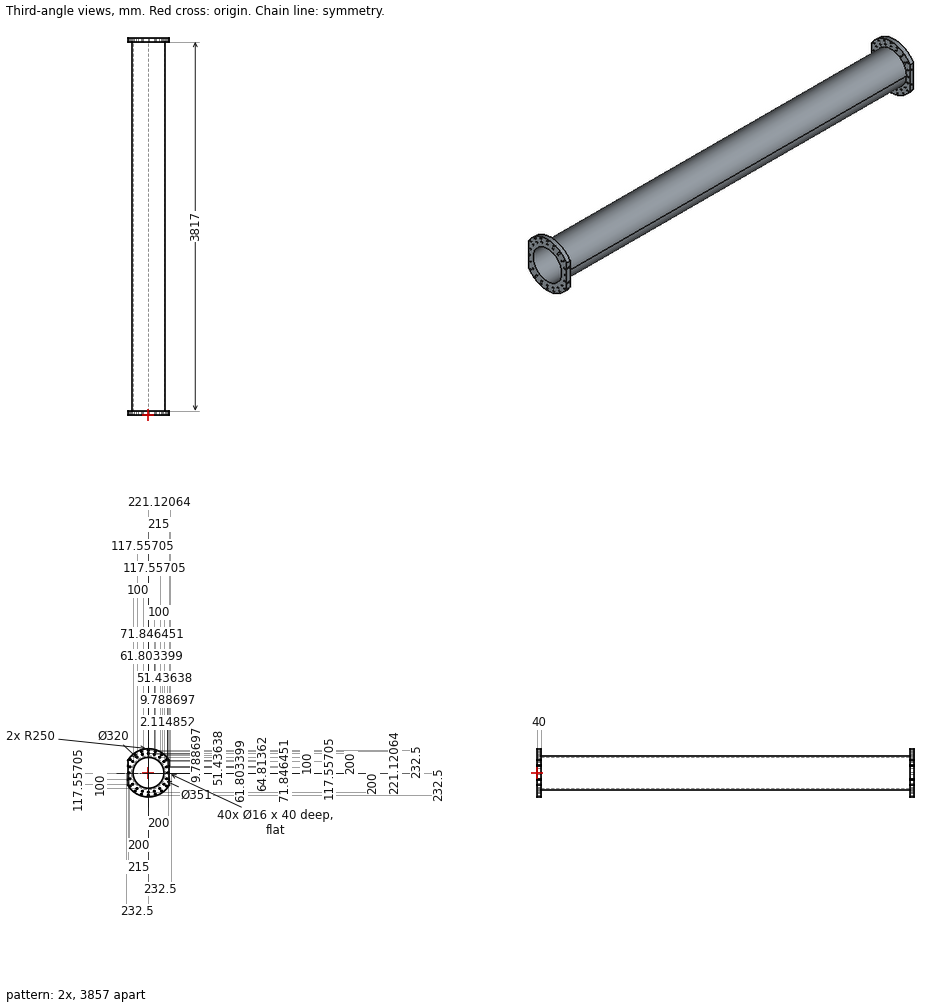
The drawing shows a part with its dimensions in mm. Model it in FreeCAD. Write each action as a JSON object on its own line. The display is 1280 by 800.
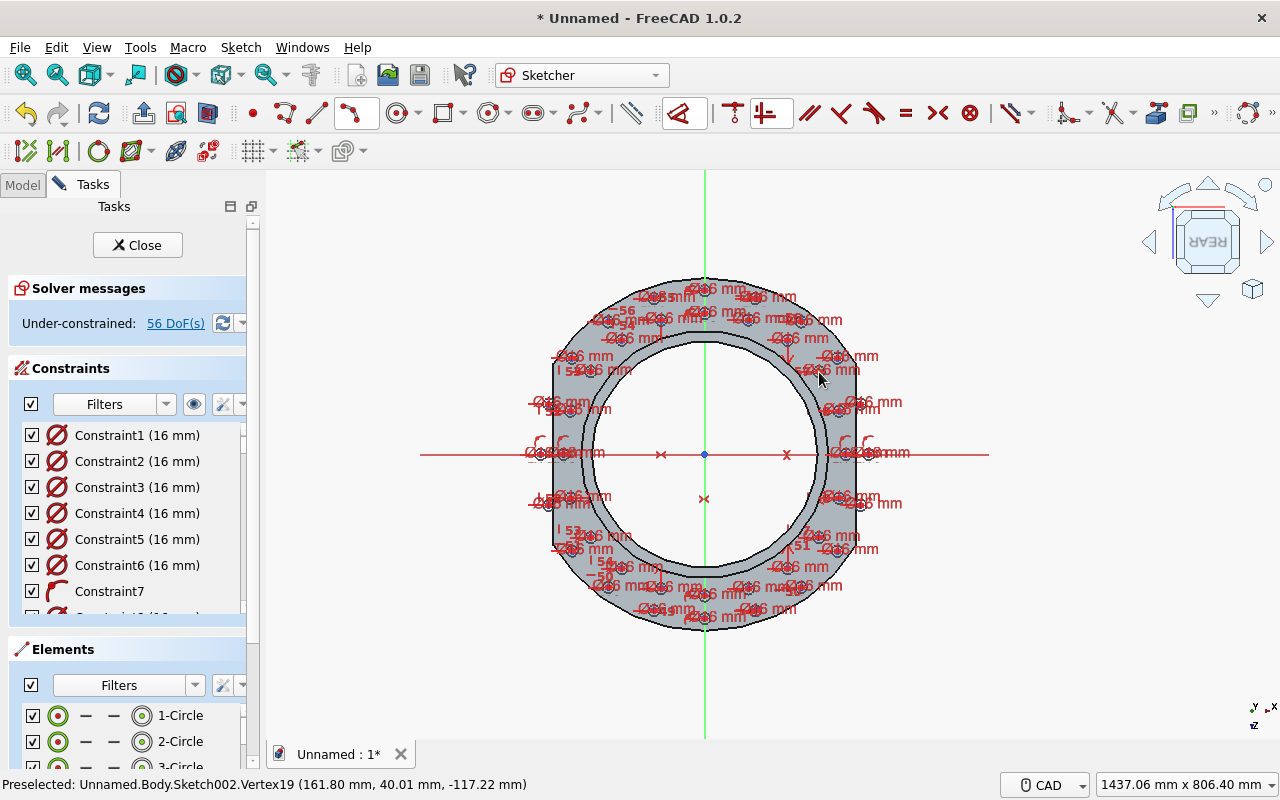
{"action": "left_click", "coordinate": [705, 674]}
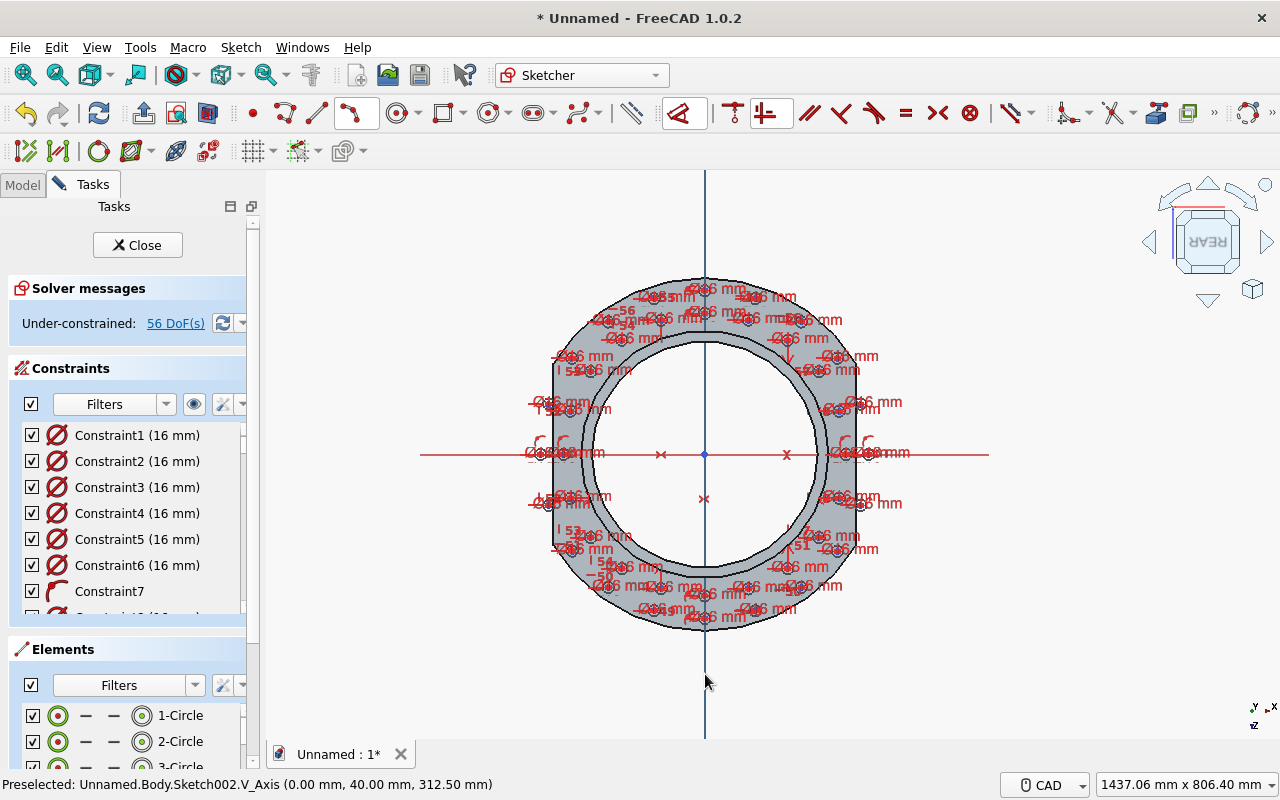
{"action": "left_click", "coordinate": [938, 114]}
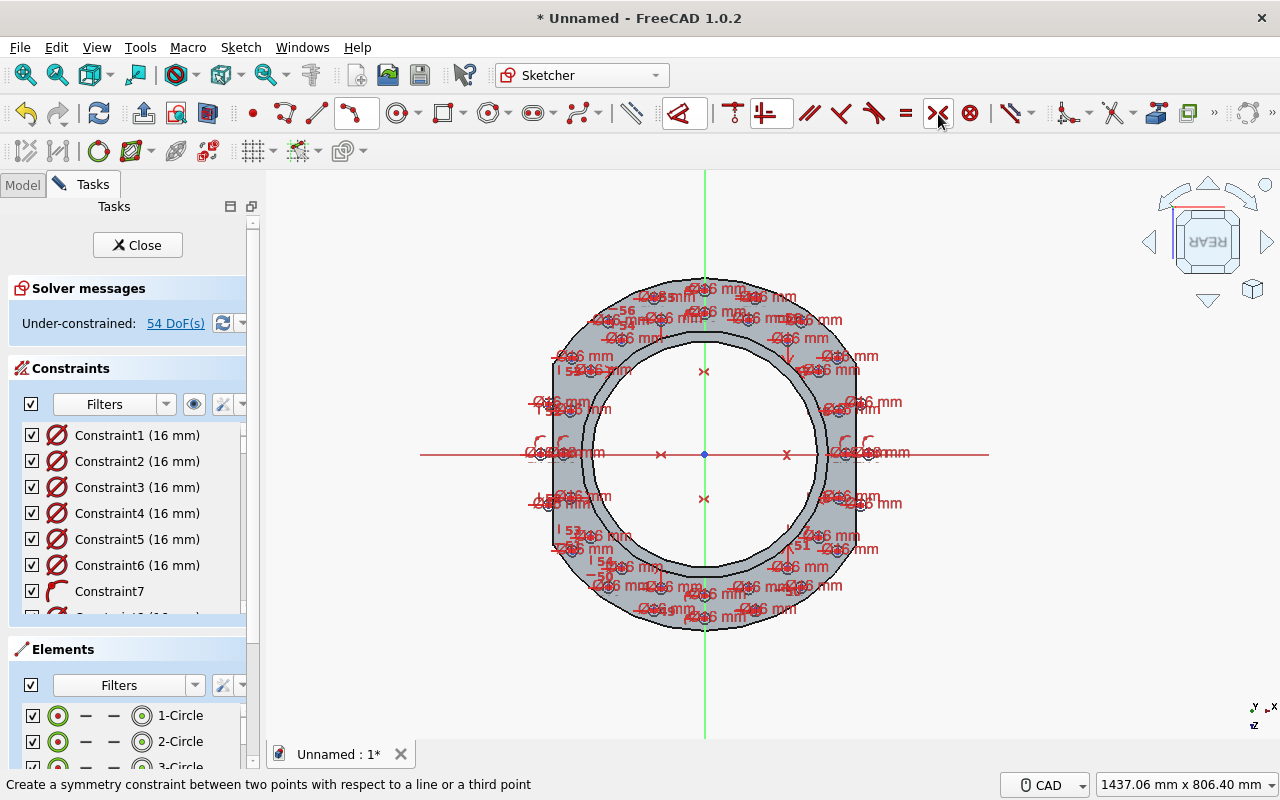
{"action": "left_click", "coordinate": [755, 611]}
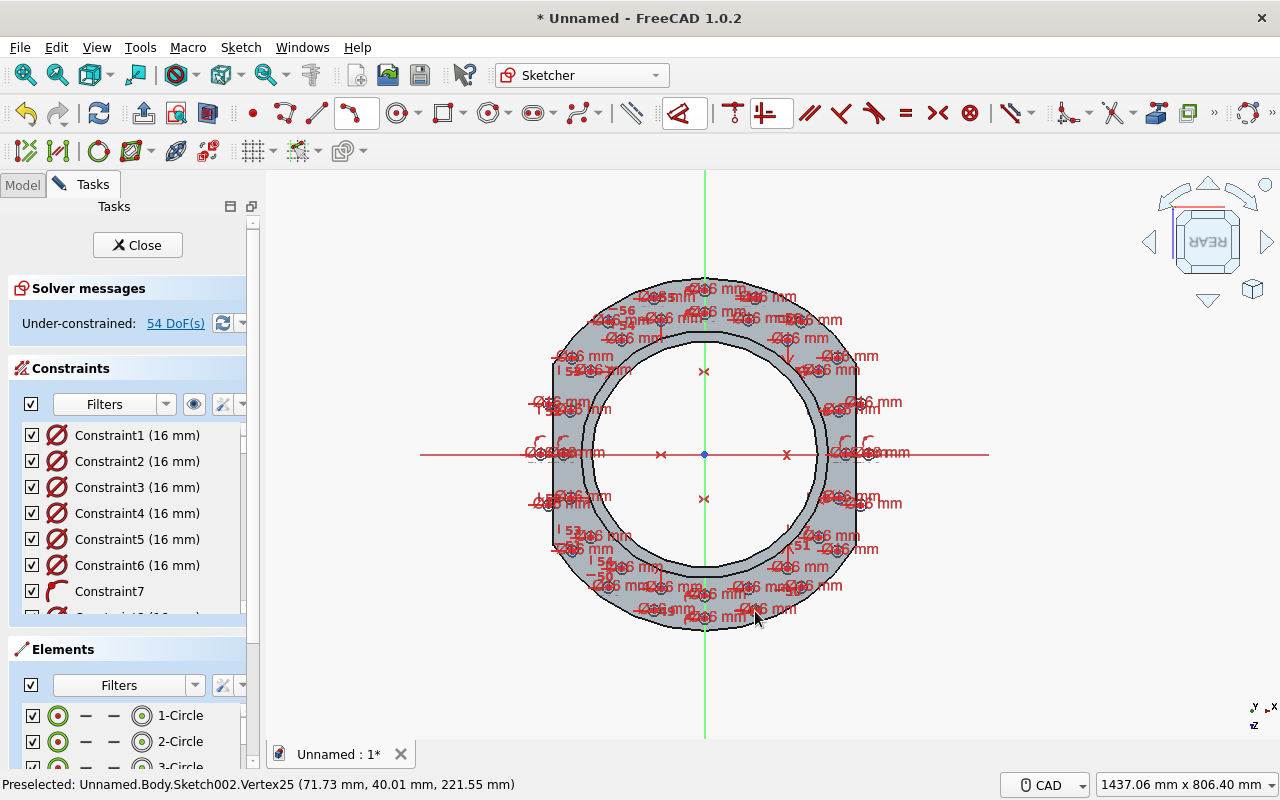
{"action": "scroll", "coordinate": [654, 611], "scroll_direction": "up", "scroll_amount": 4}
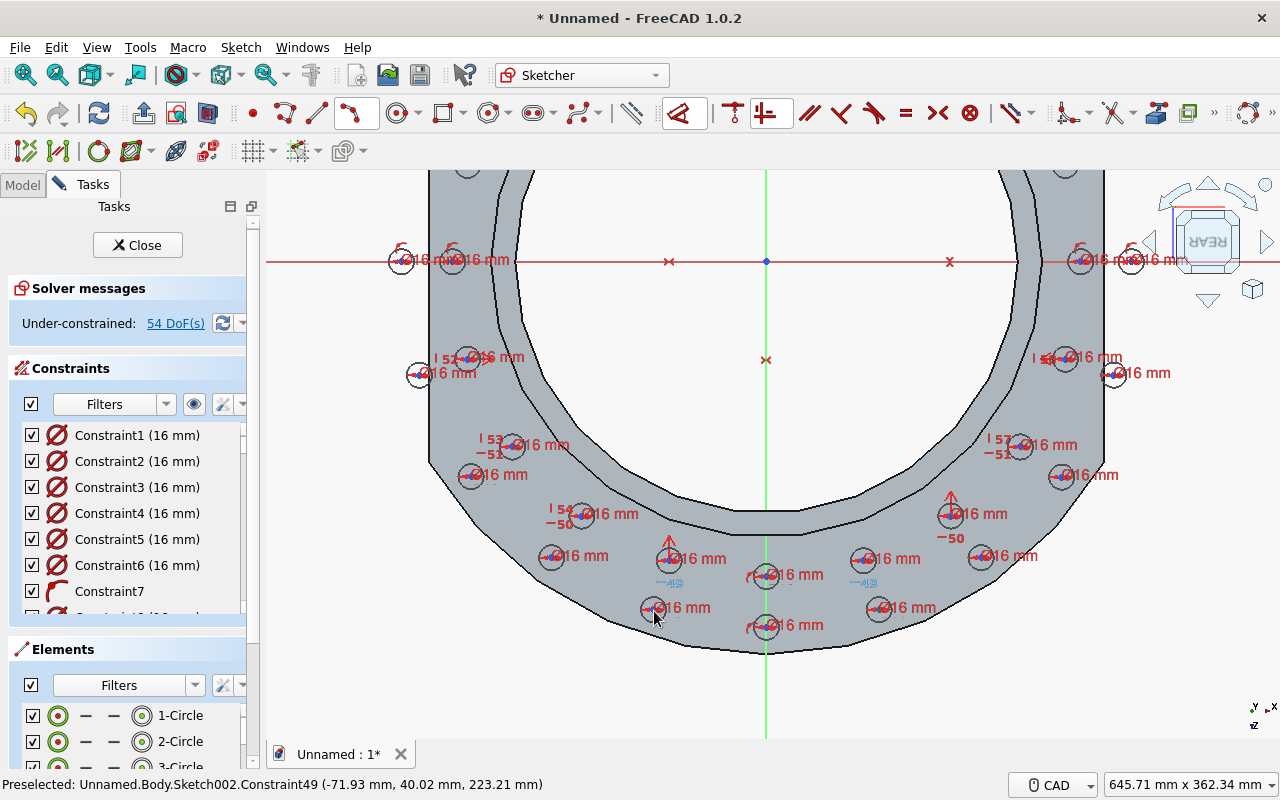
{"action": "left_click", "coordinate": [654, 610]}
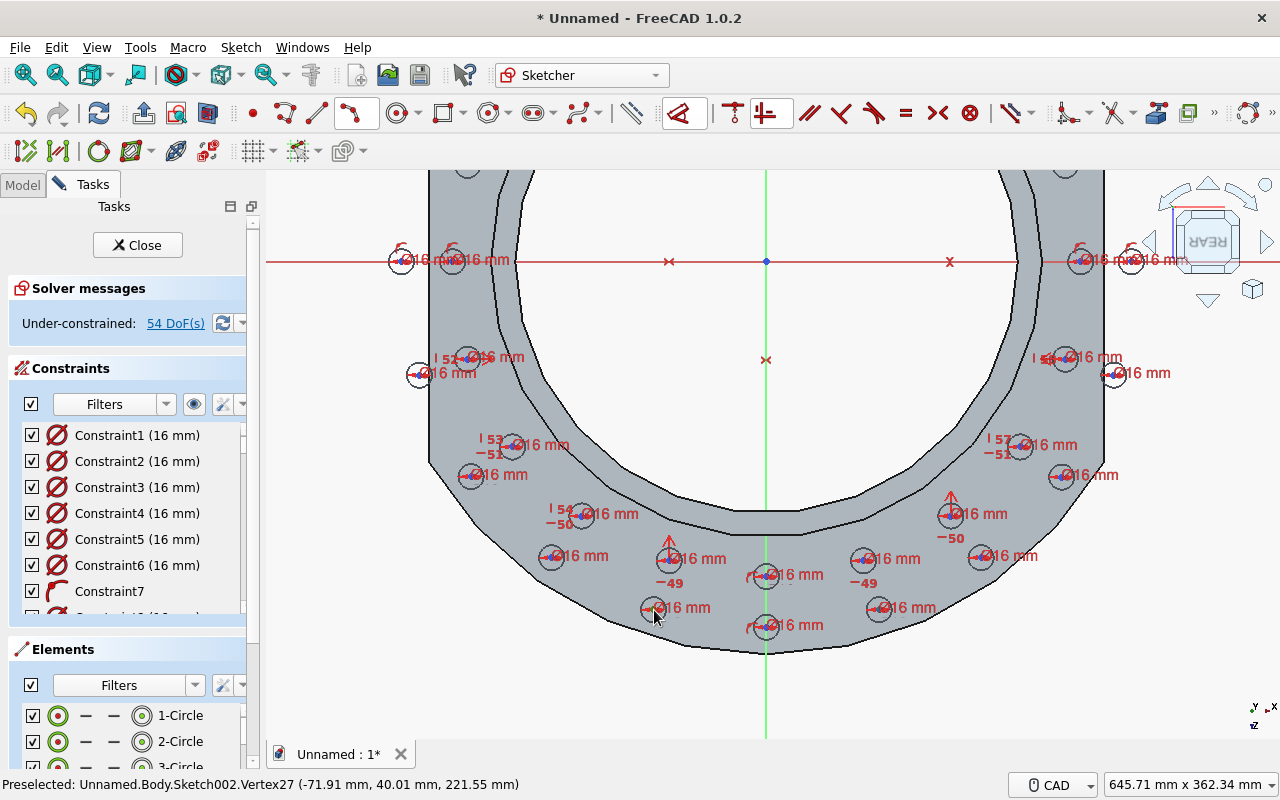
{"action": "left_click", "coordinate": [766, 674]}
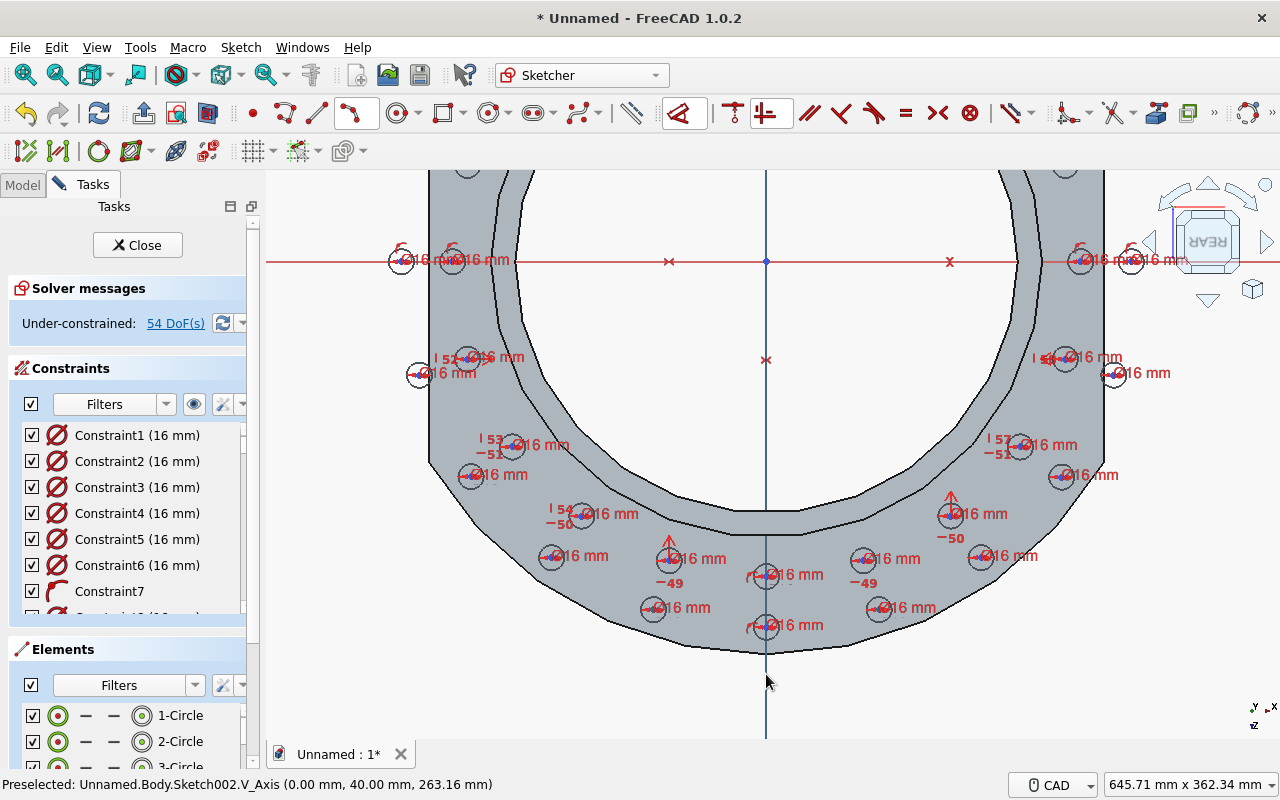
{"action": "left_click", "coordinate": [938, 114]}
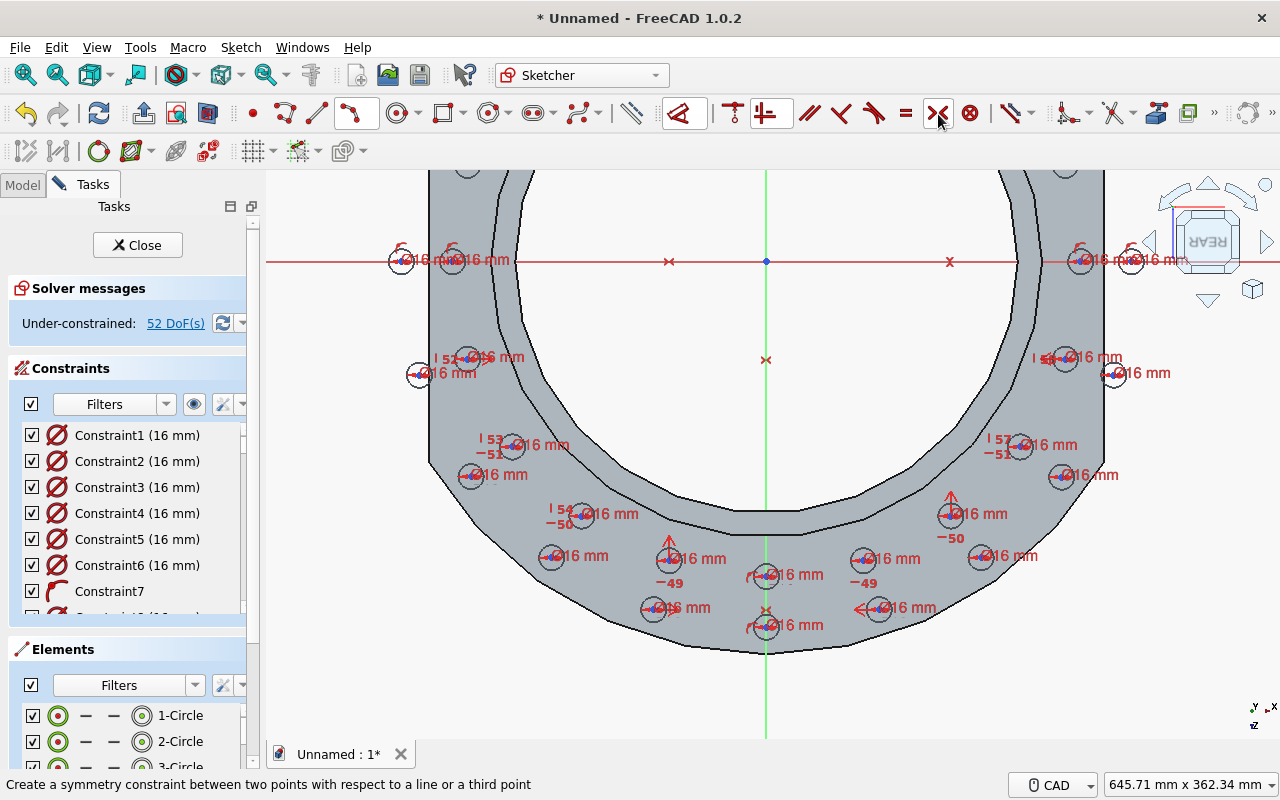
{"action": "left_click", "coordinate": [981, 558]}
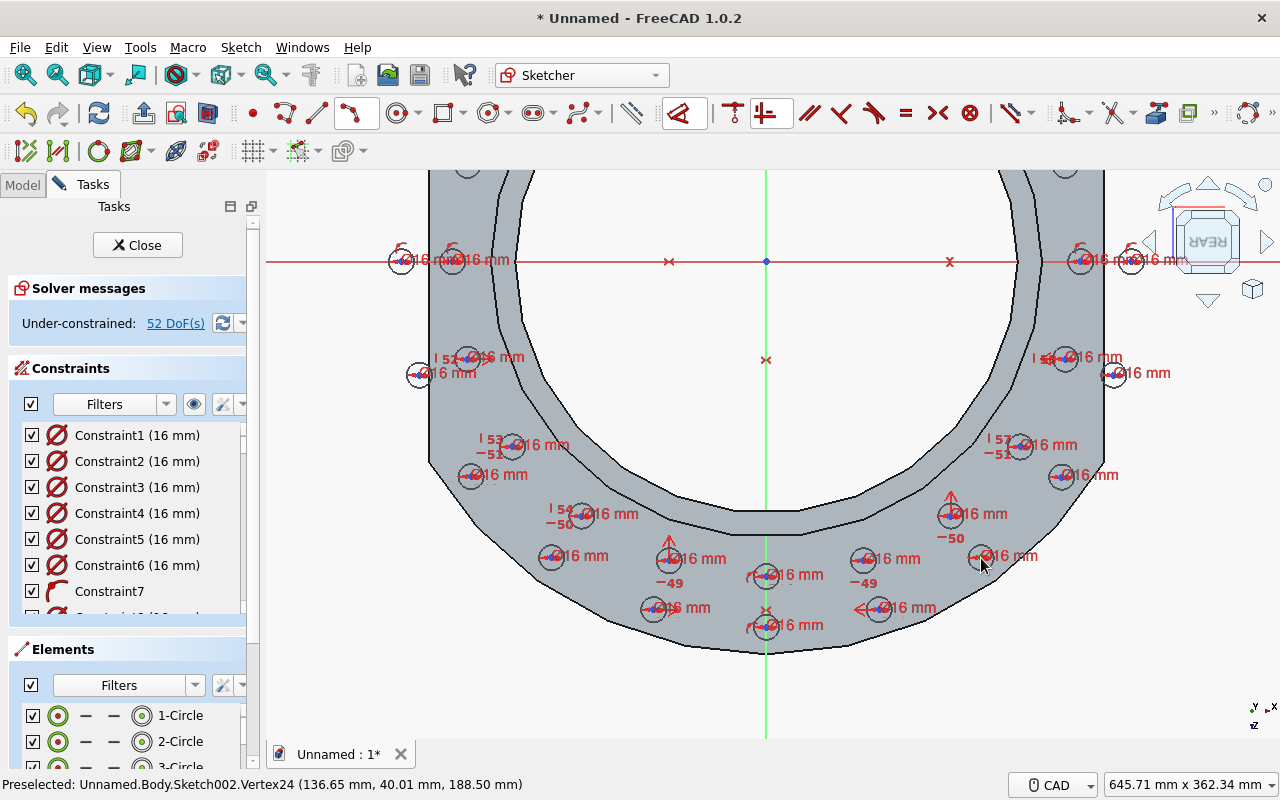
{"action": "left_click", "coordinate": [552, 558]}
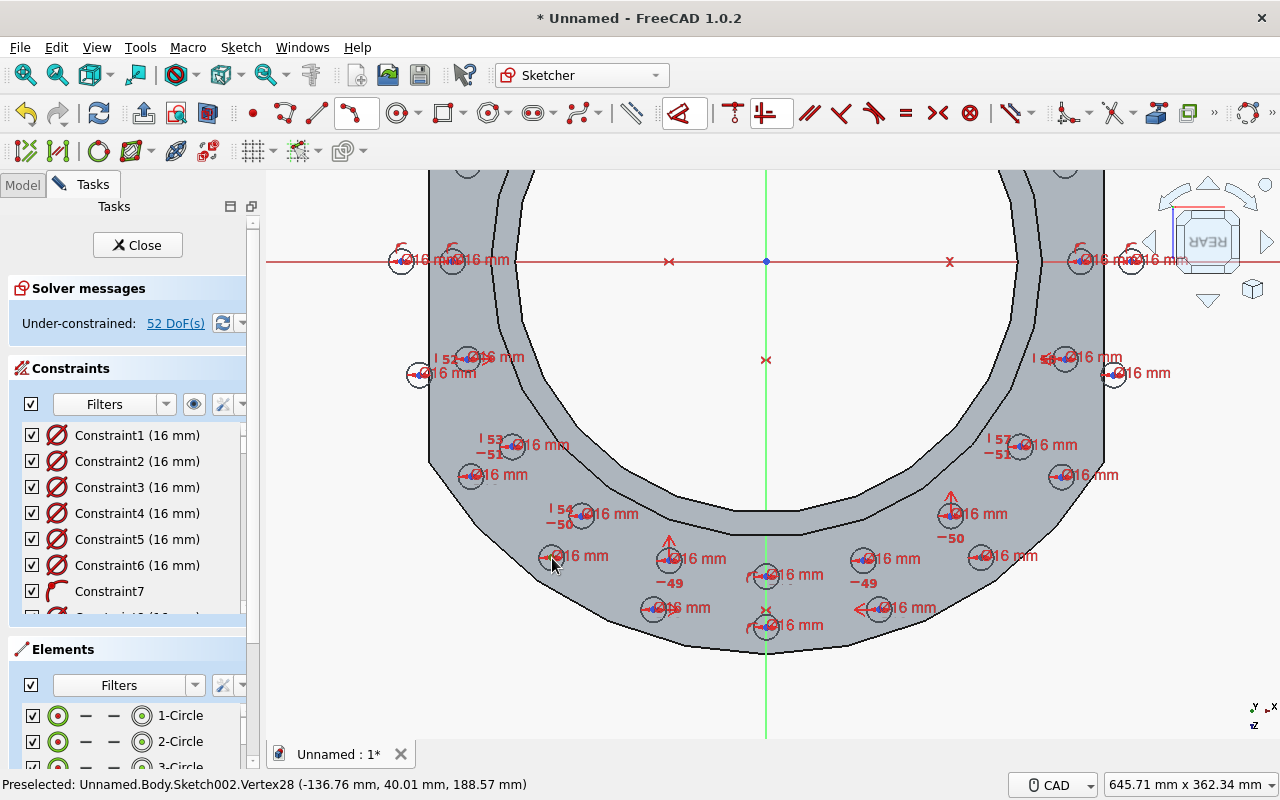
{"action": "left_click", "coordinate": [766, 674]}